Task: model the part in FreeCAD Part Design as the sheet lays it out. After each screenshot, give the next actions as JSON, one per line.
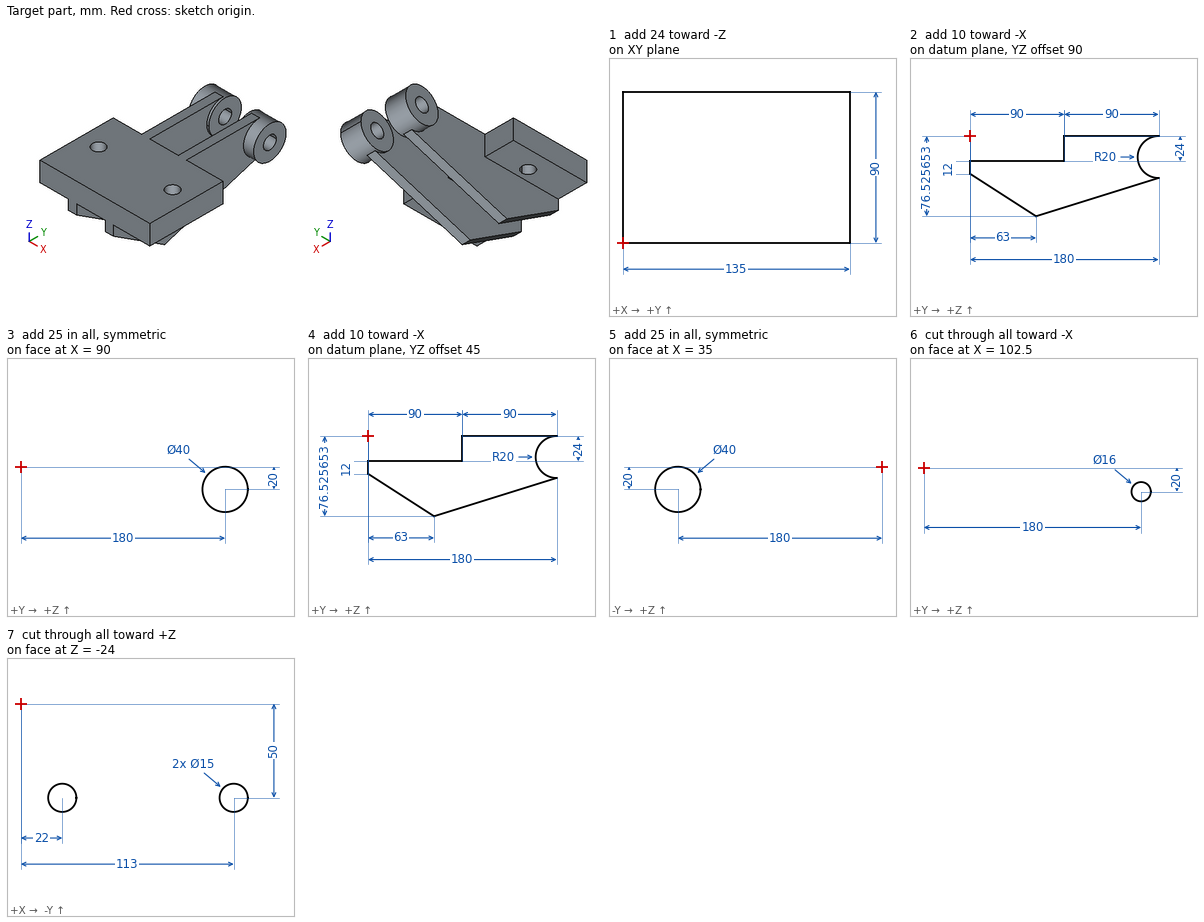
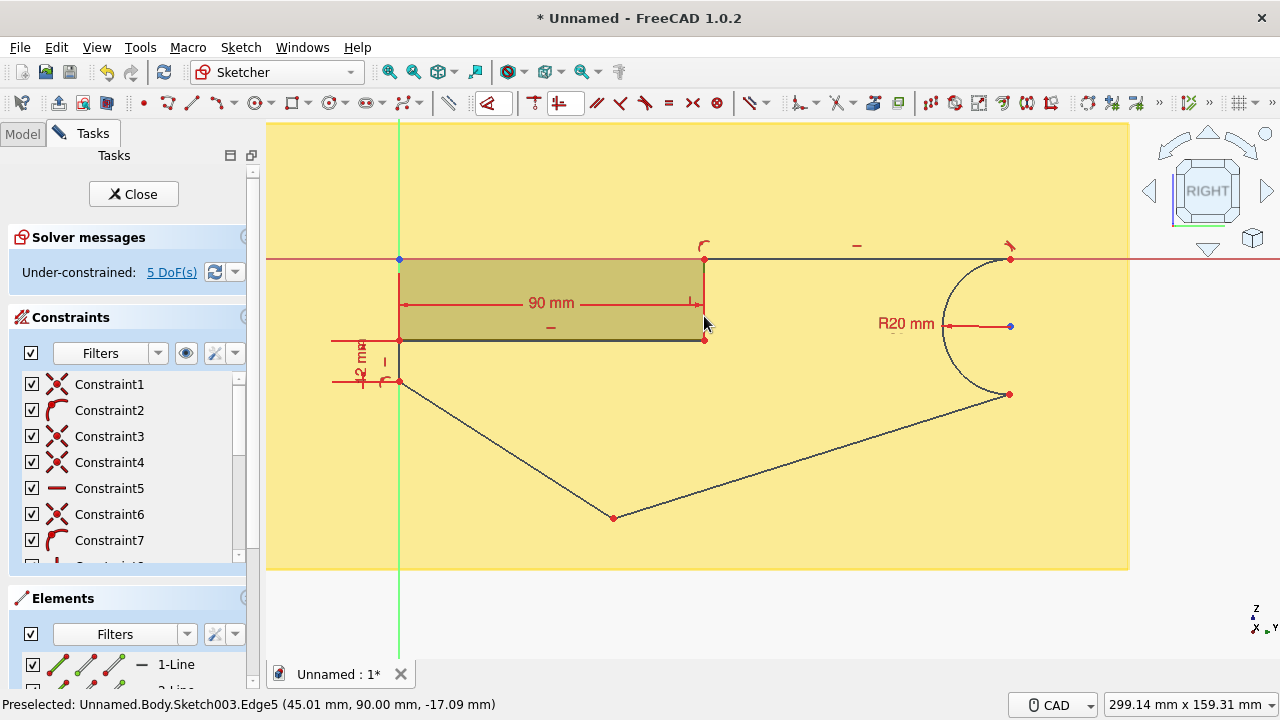
{"action": "key", "text": "i"}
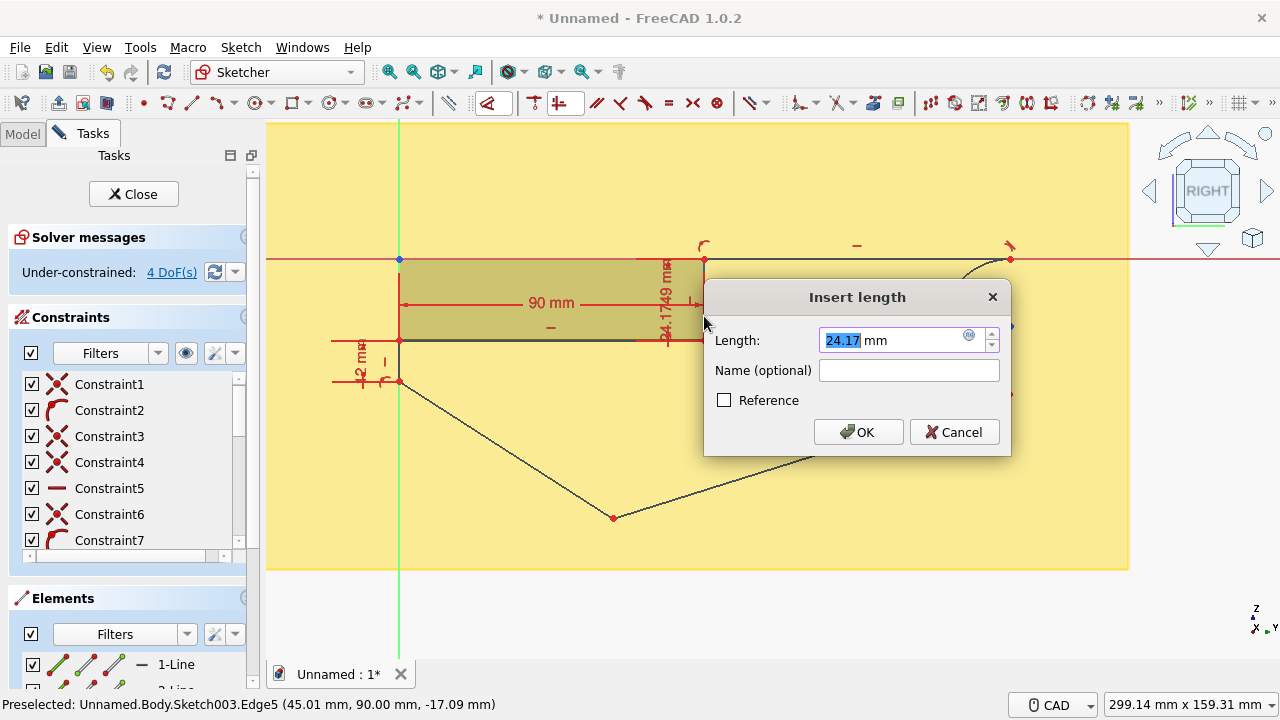
{"action": "type", "text": "24"}
{"action": "key", "text": "Return"}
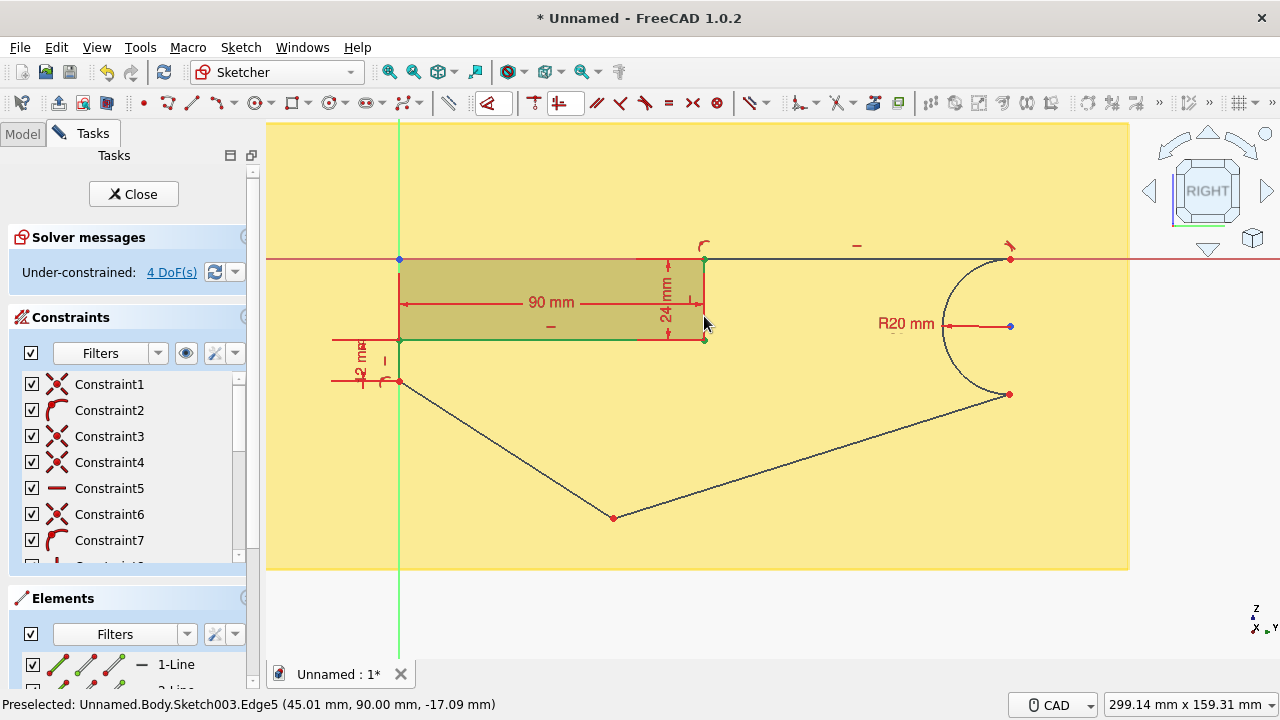
{"action": "left_click", "coordinate": [796, 259]}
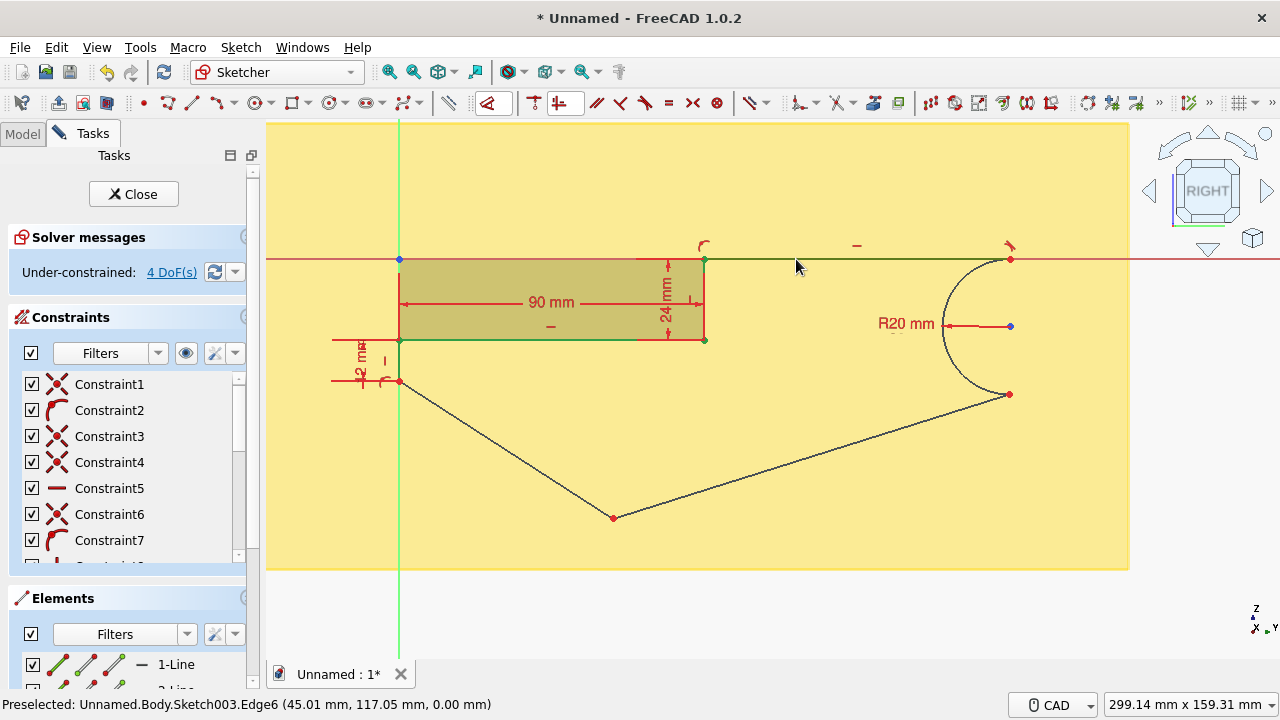
{"action": "key", "text": "l"}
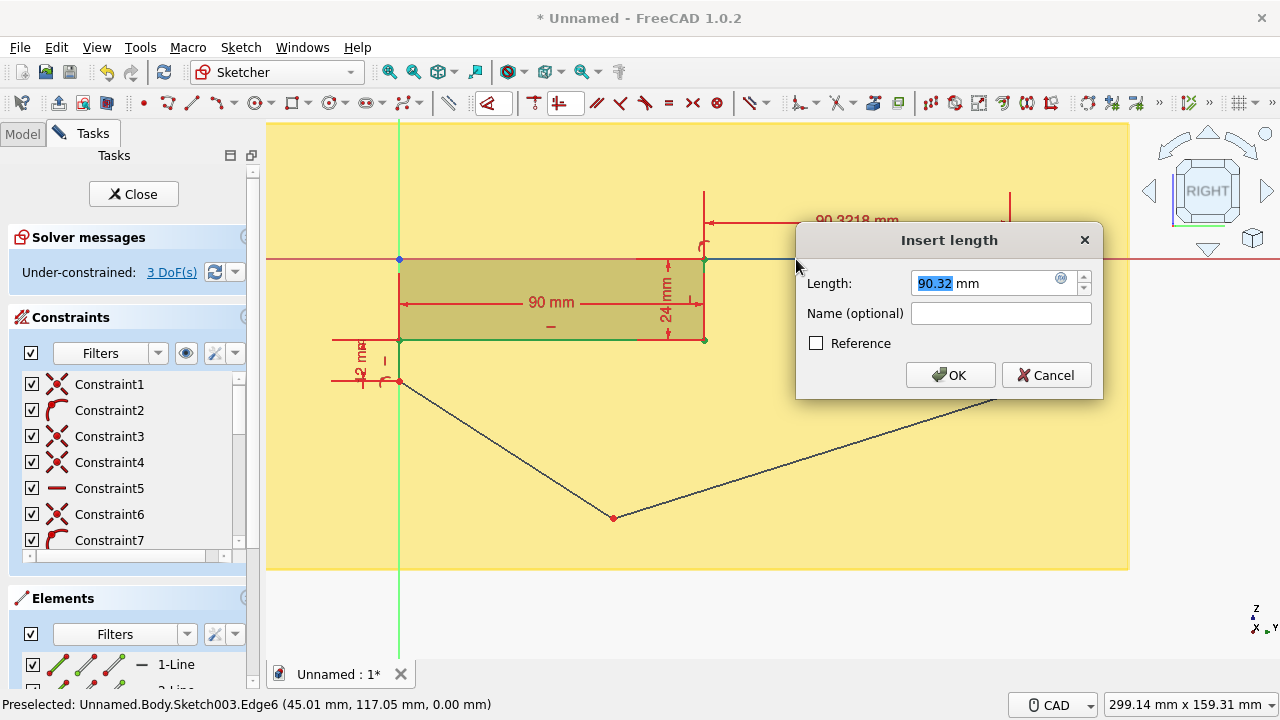
{"action": "type", "text": "90"}
{"action": "key", "text": "Return"}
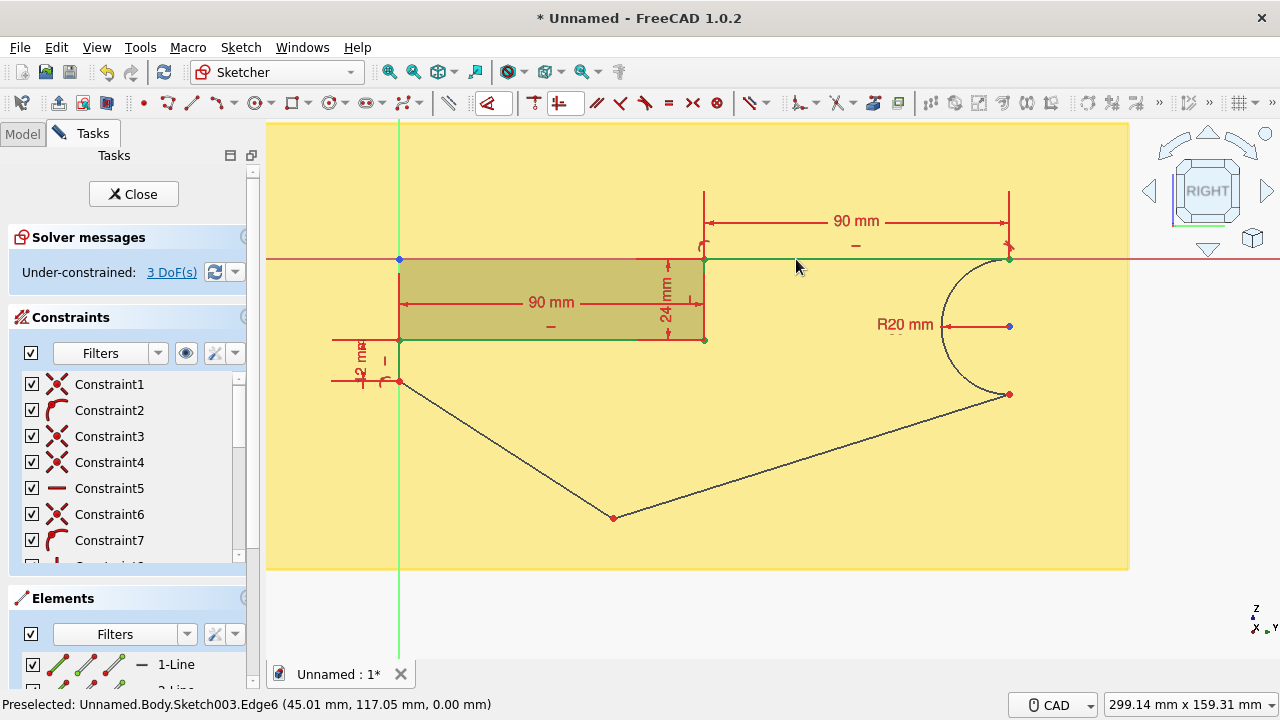
{"action": "left_click", "coordinate": [613, 519]}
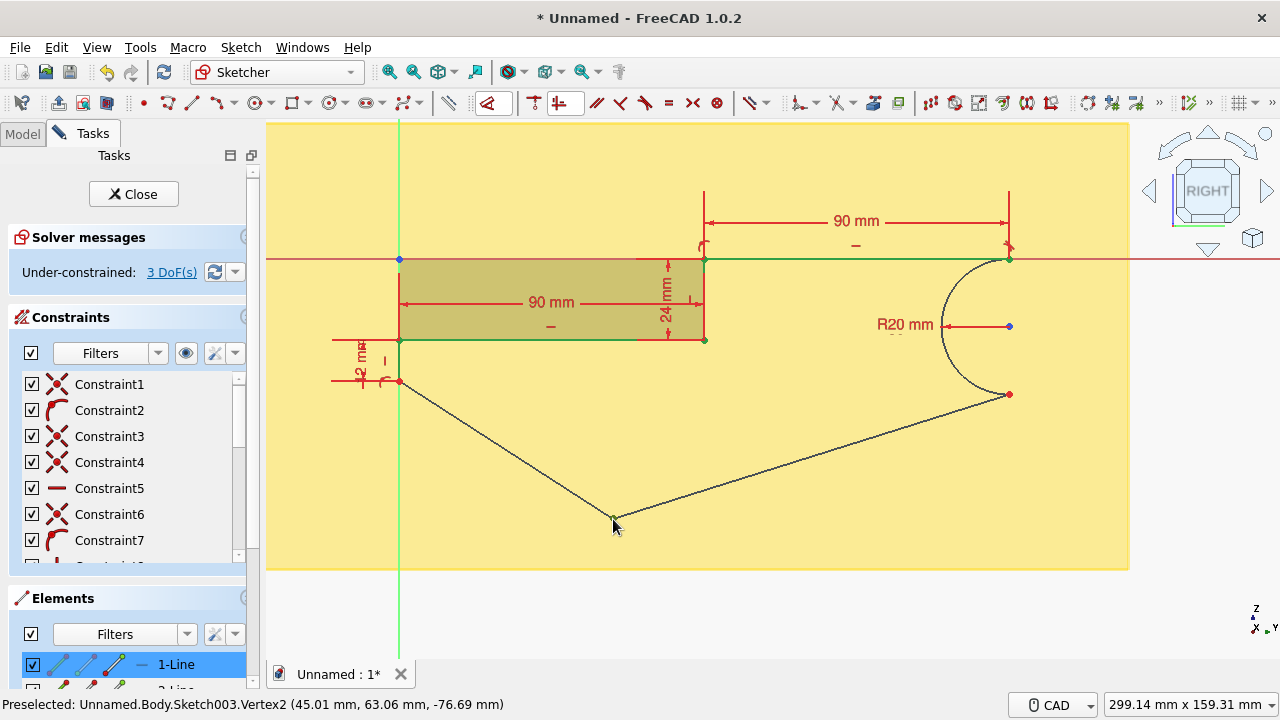
{"action": "key", "text": "l"}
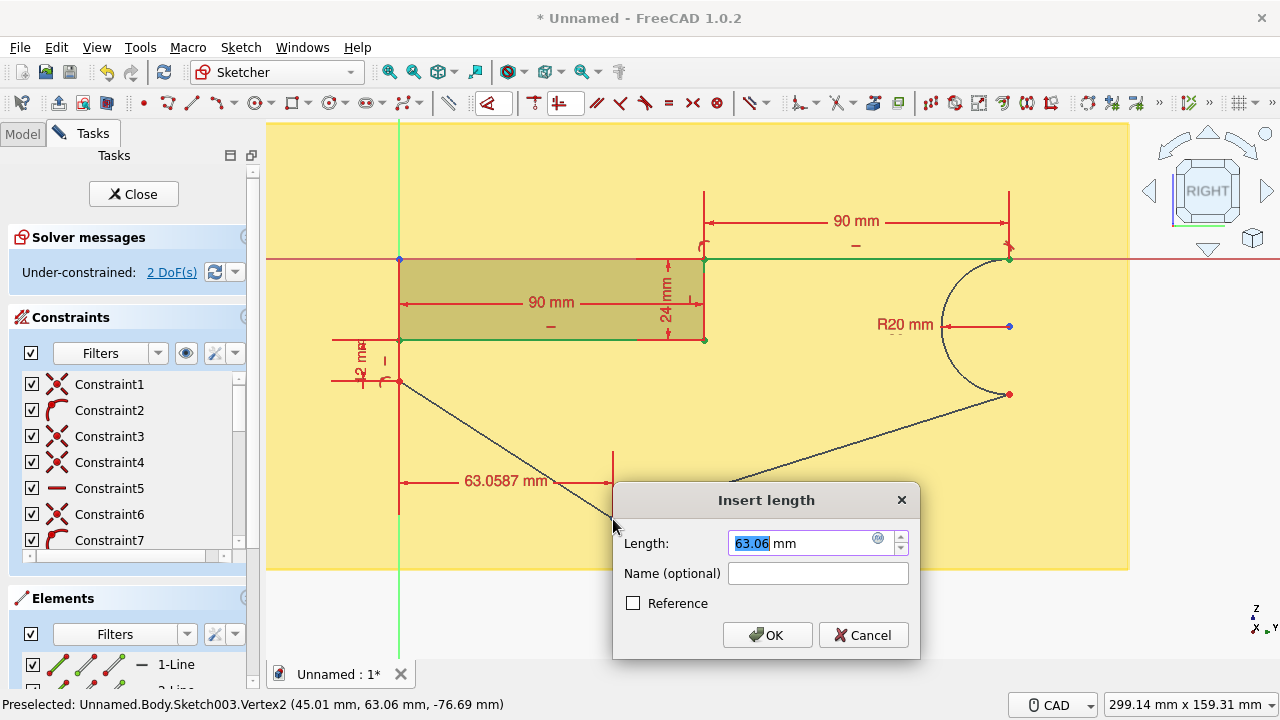
{"action": "type", "text": "63"}
{"action": "key", "text": "Return"}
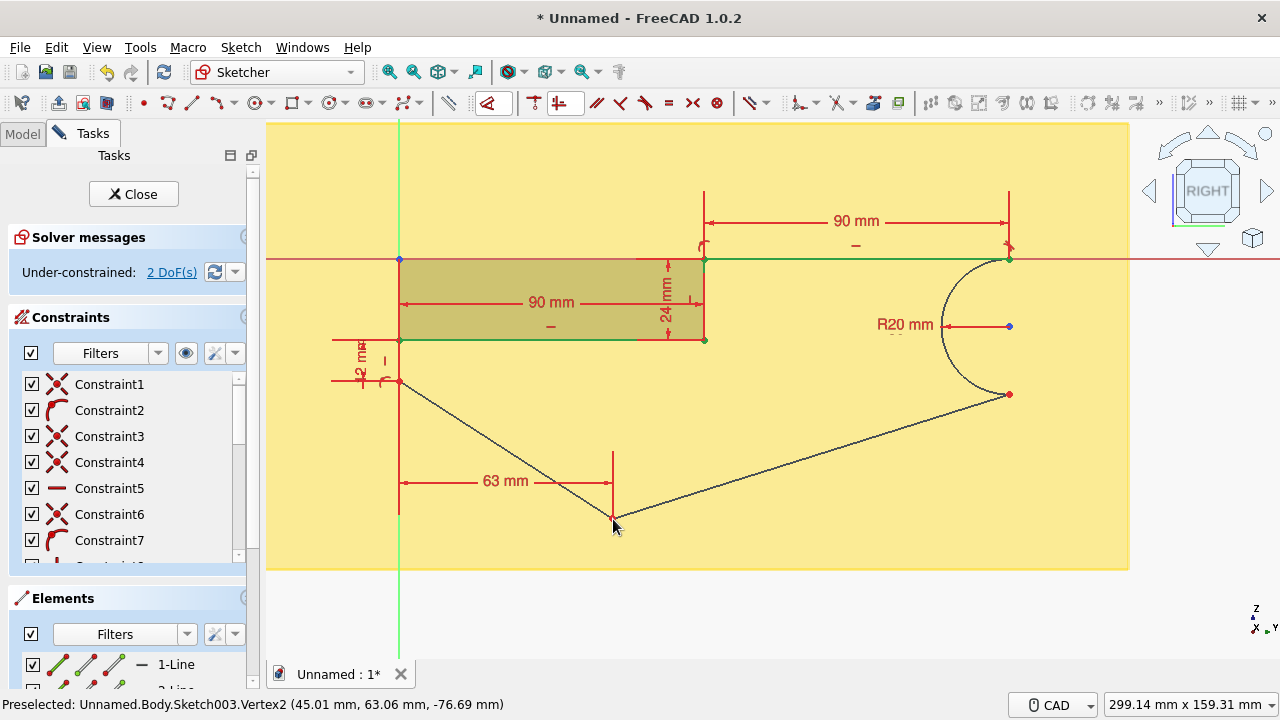
{"action": "left_click", "coordinate": [1009, 395]}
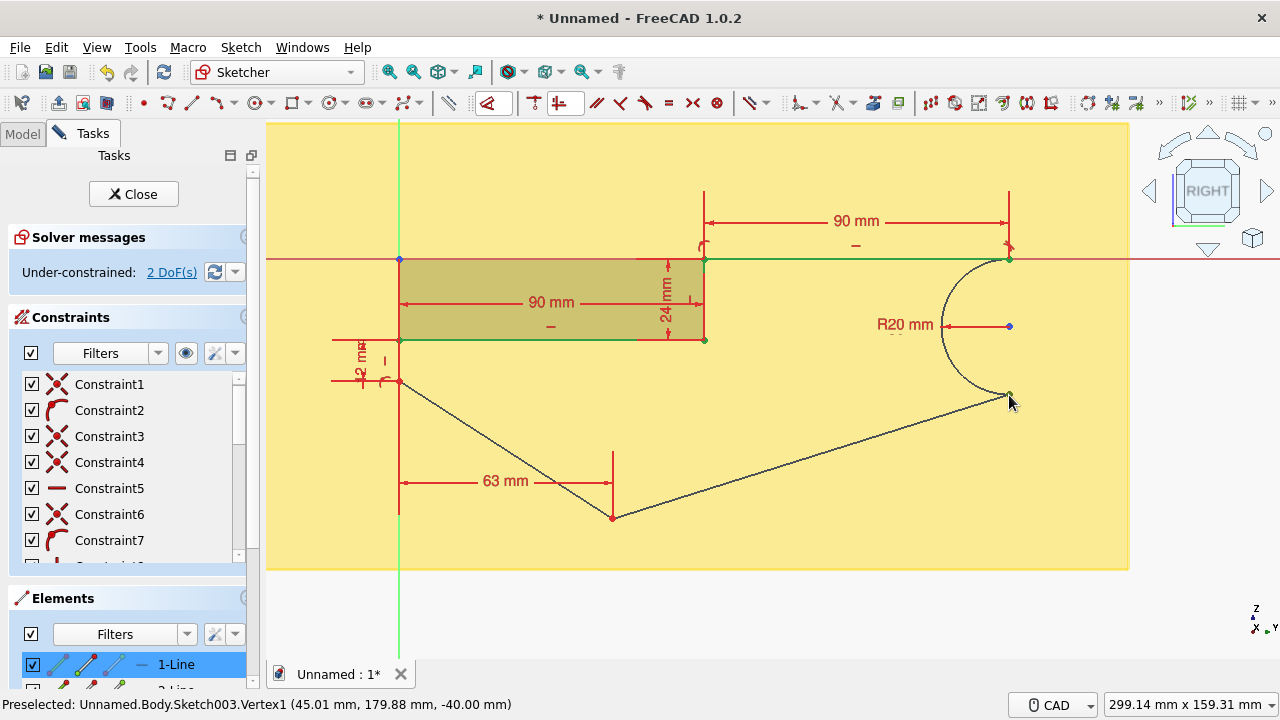
{"action": "key", "text": "l"}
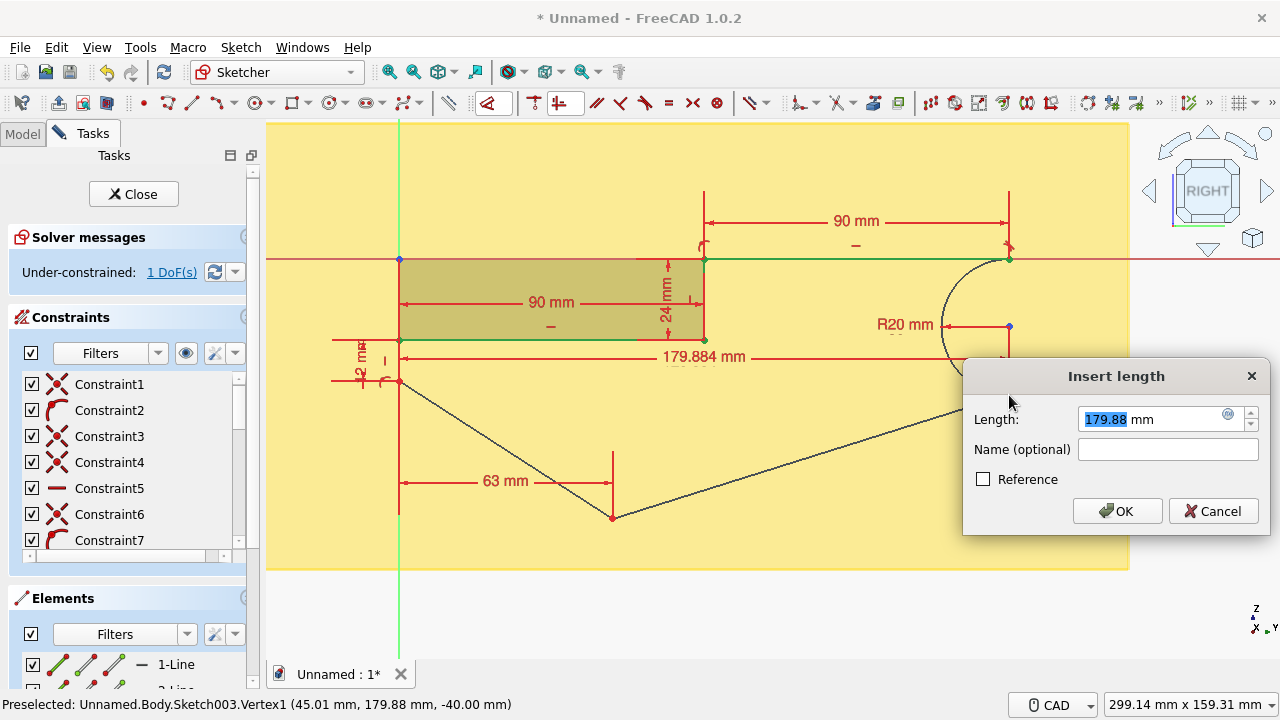
{"action": "type", "text": "180"}
{"action": "key", "text": "Return"}